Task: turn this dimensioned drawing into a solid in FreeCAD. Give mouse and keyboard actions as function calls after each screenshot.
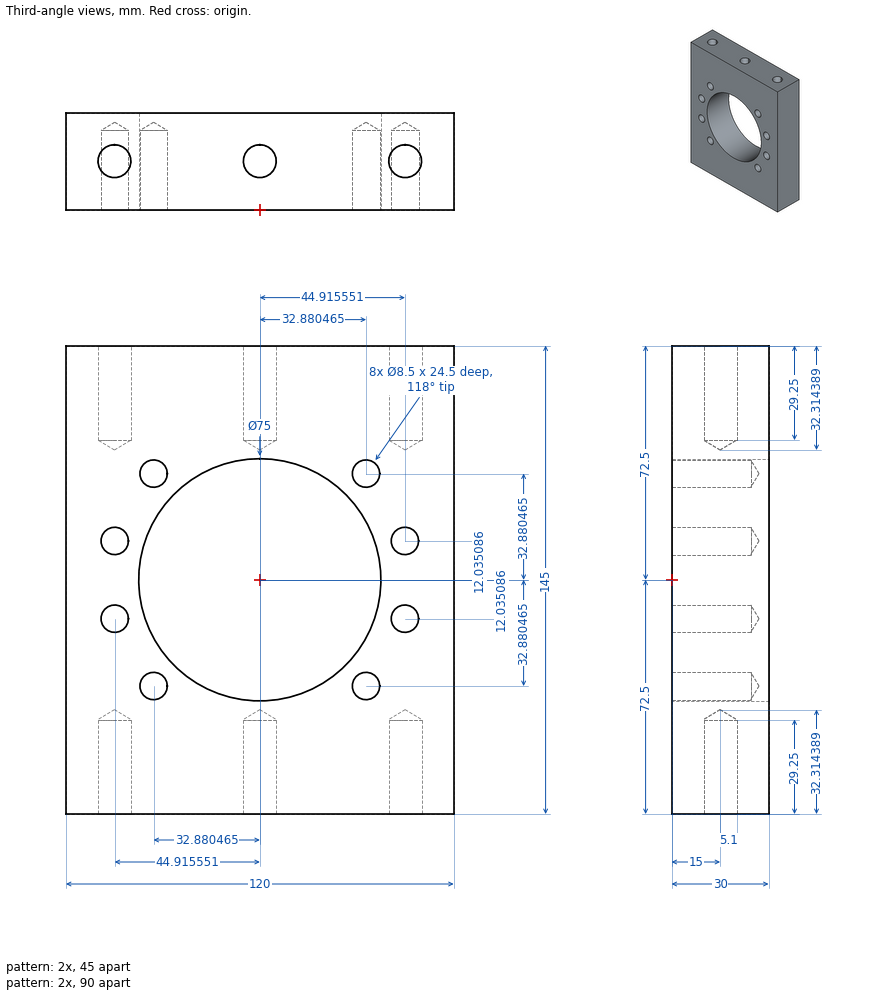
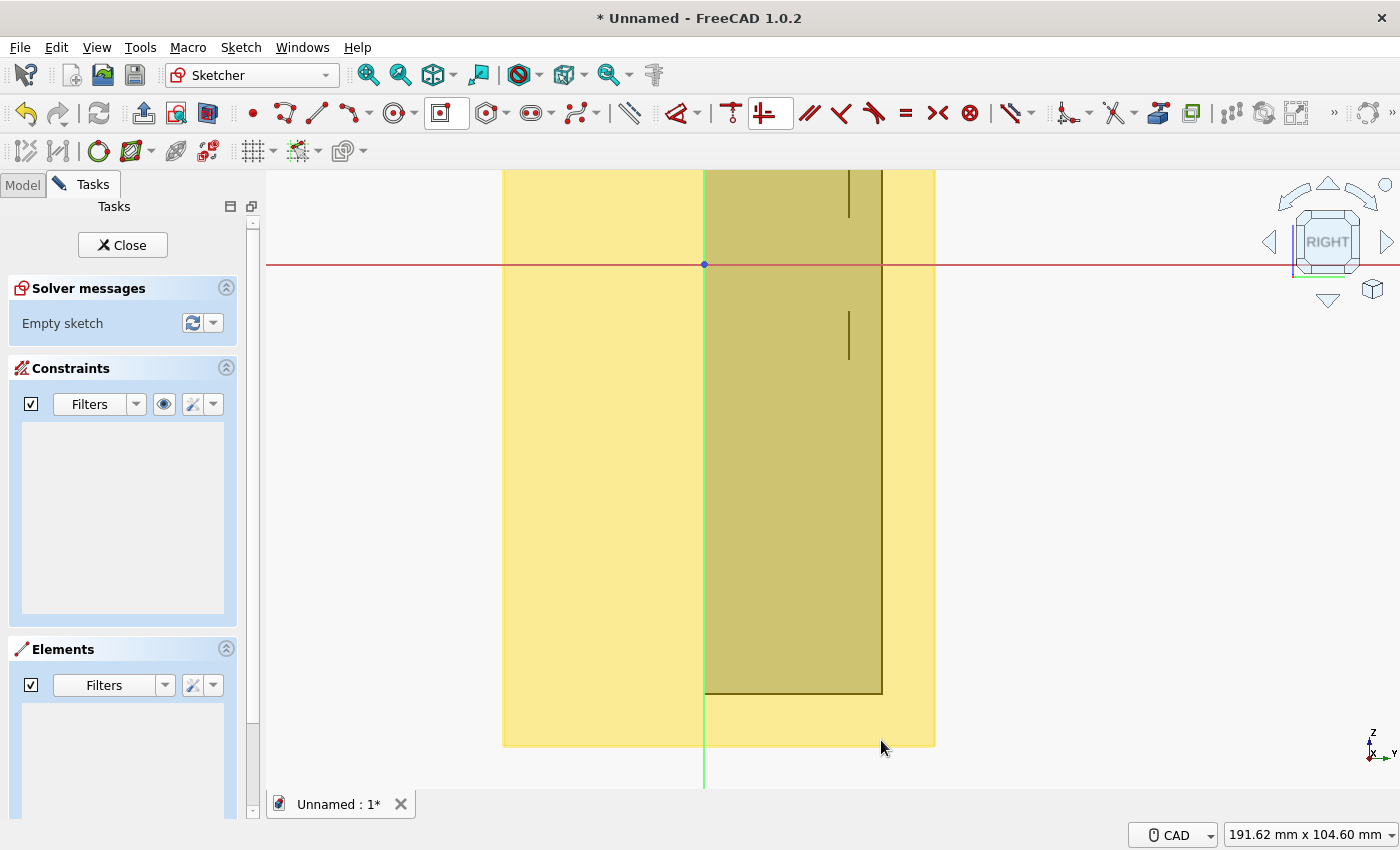
click(286, 114)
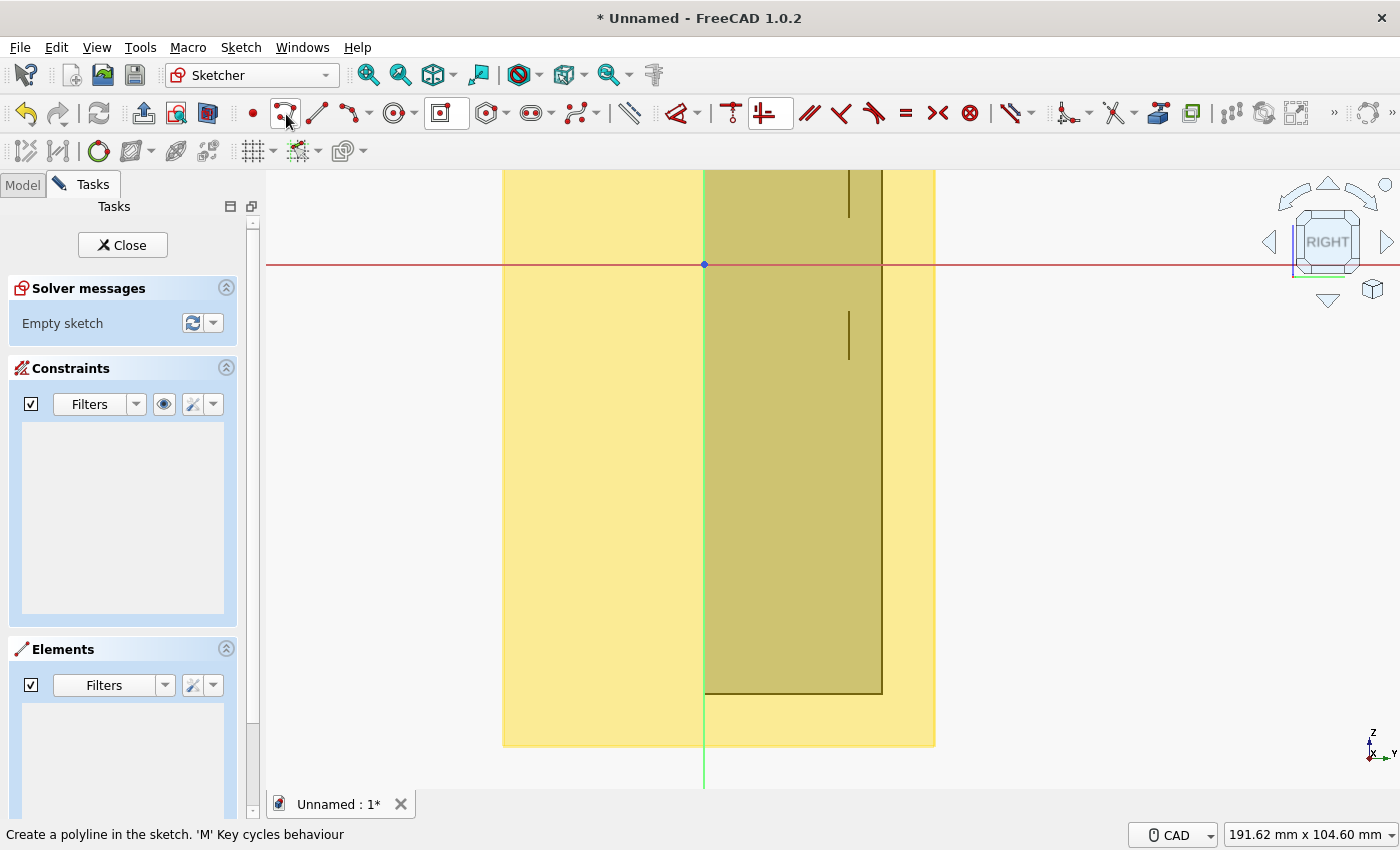
click(793, 502)
click(793, 694)
click(823, 694)
click(823, 521)
click(793, 503)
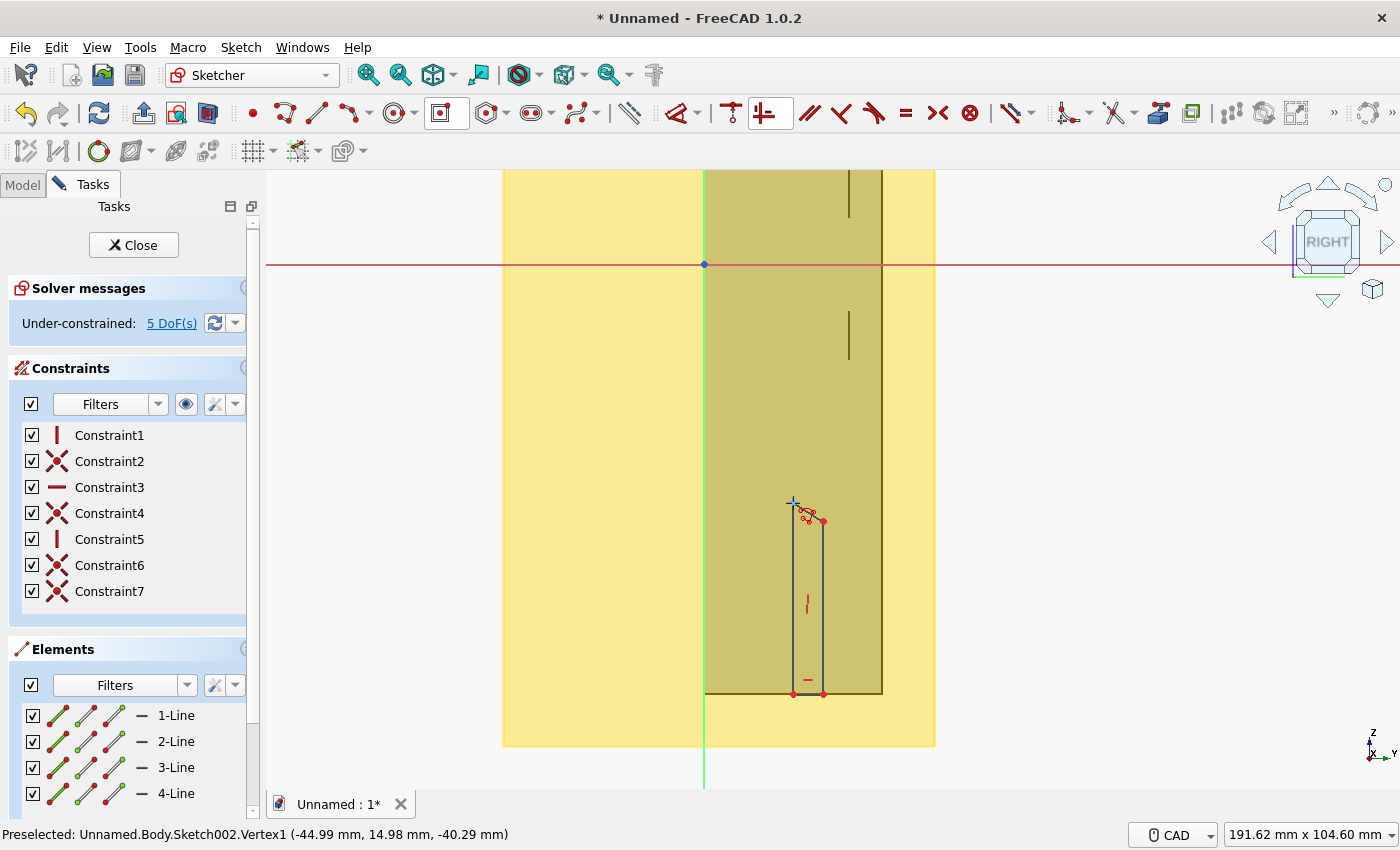
click(318, 114)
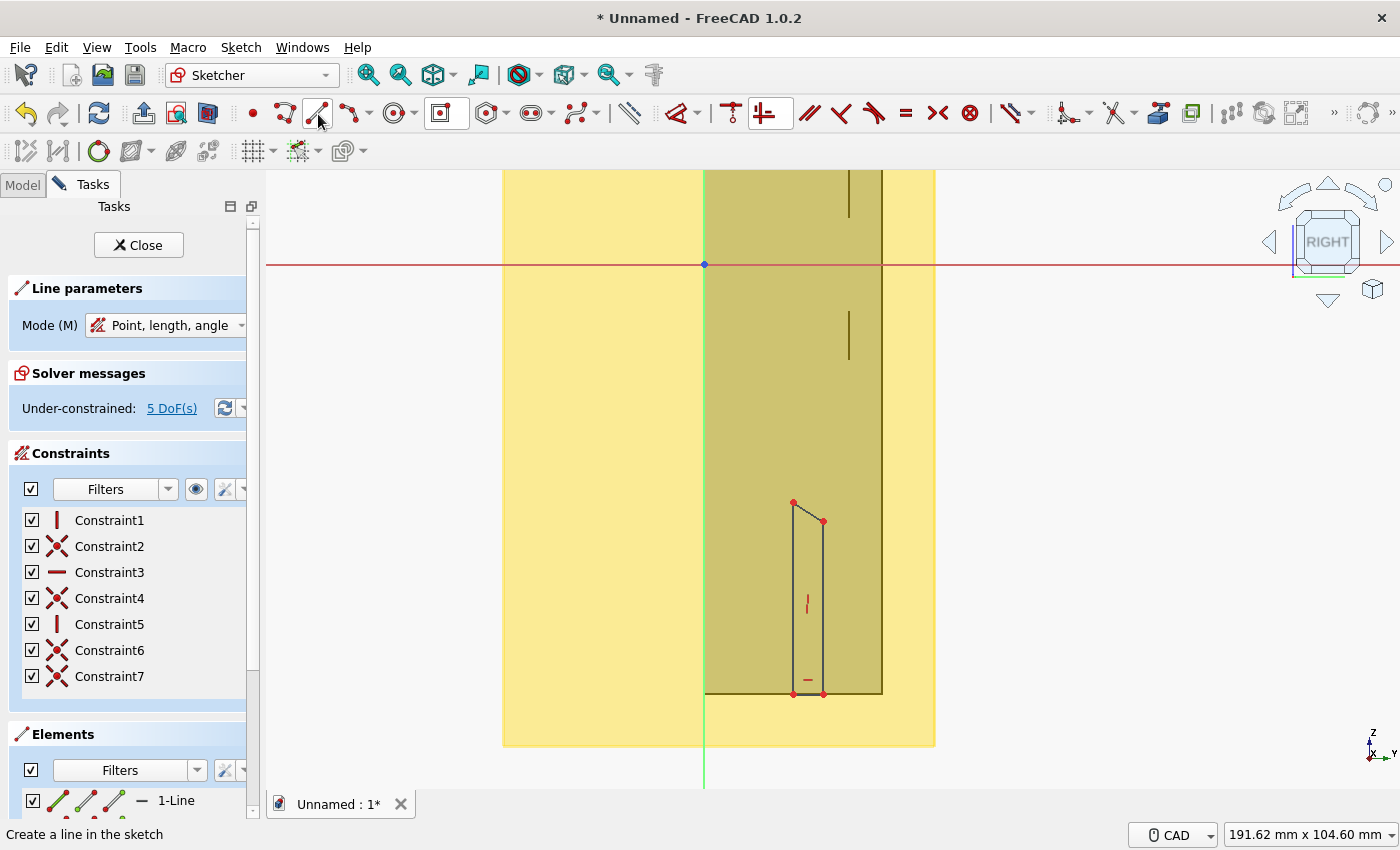
click(793, 483)
click(793, 426)
key(Escape)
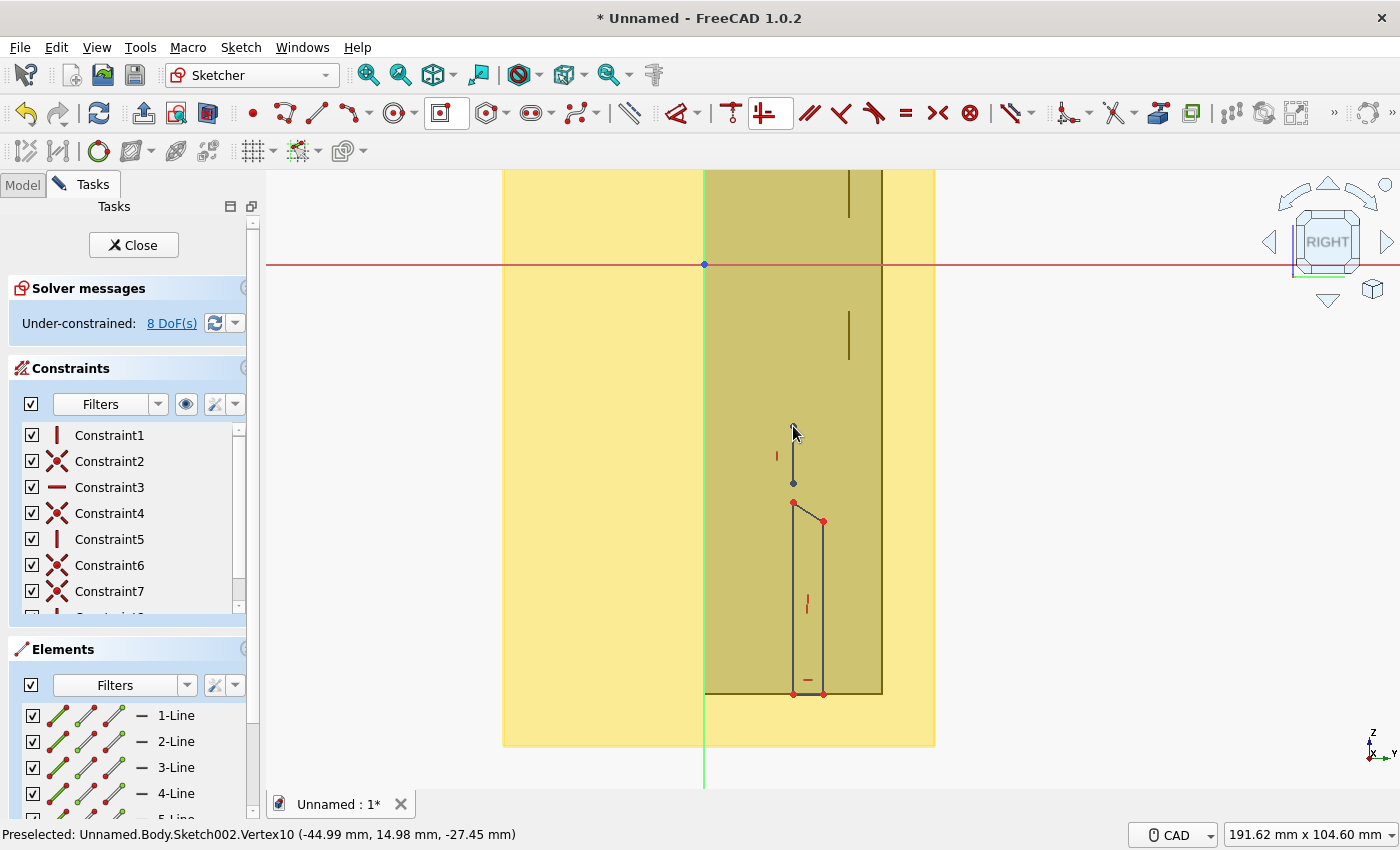
click(793, 467)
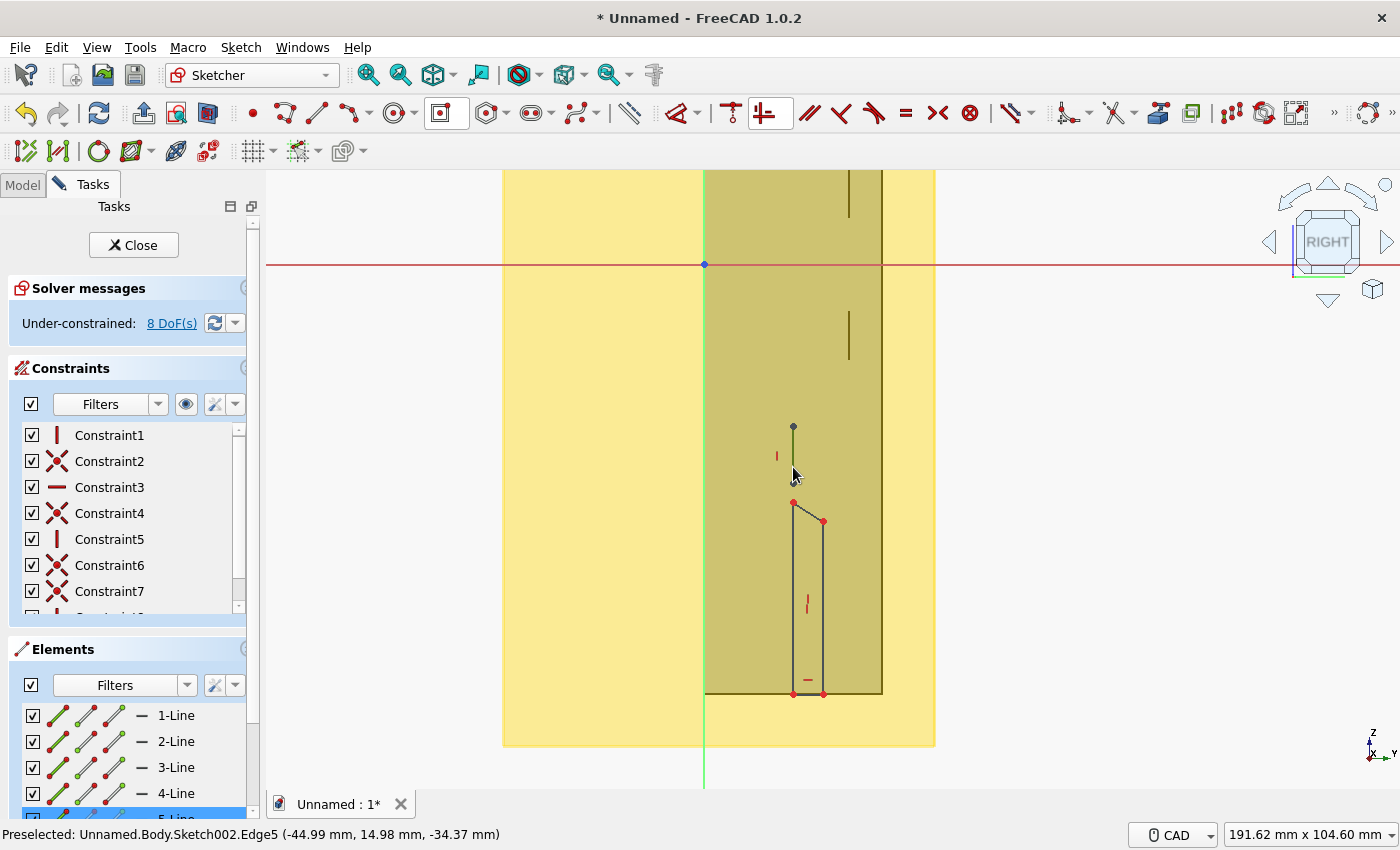
click(630, 114)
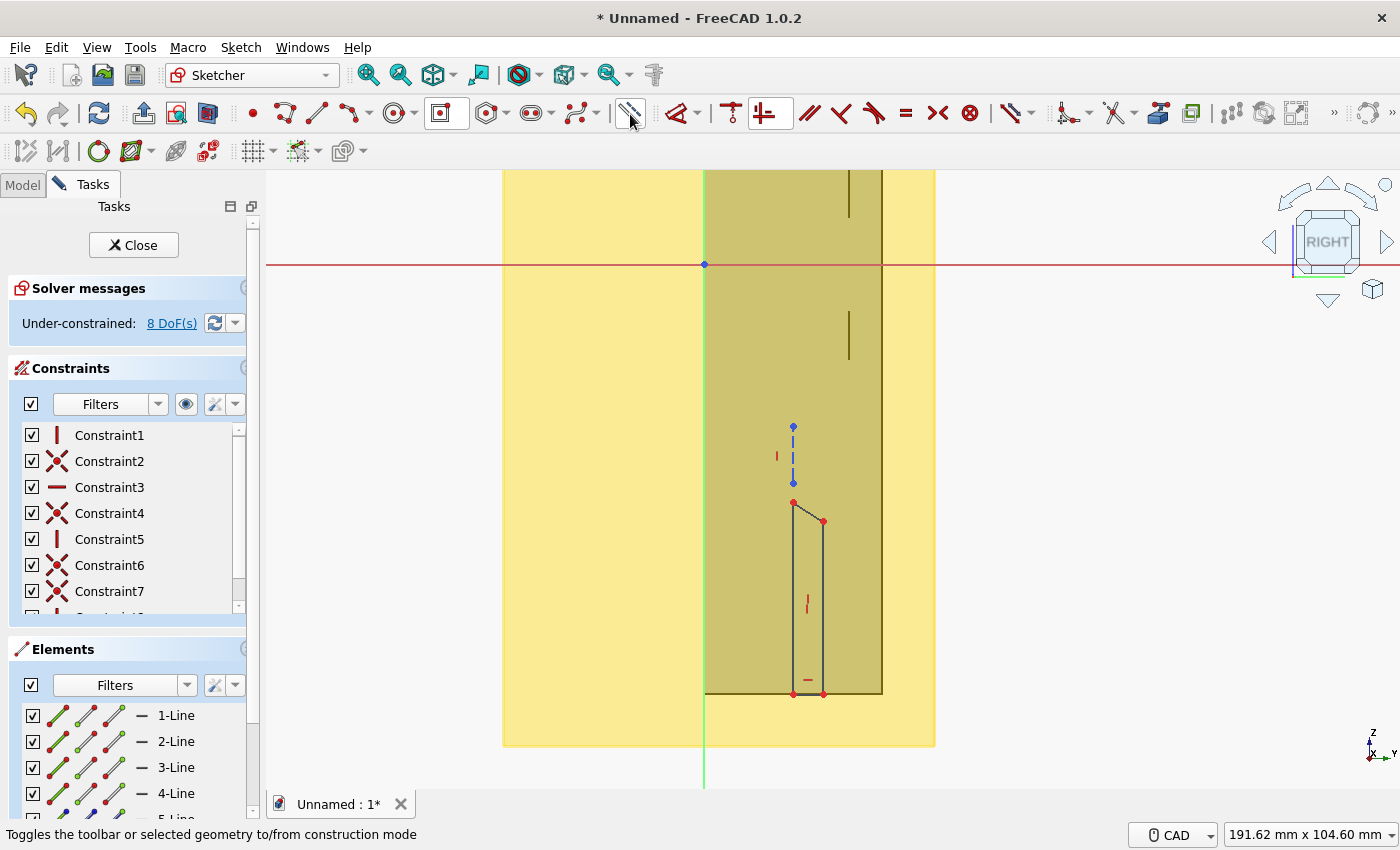
click(676, 114)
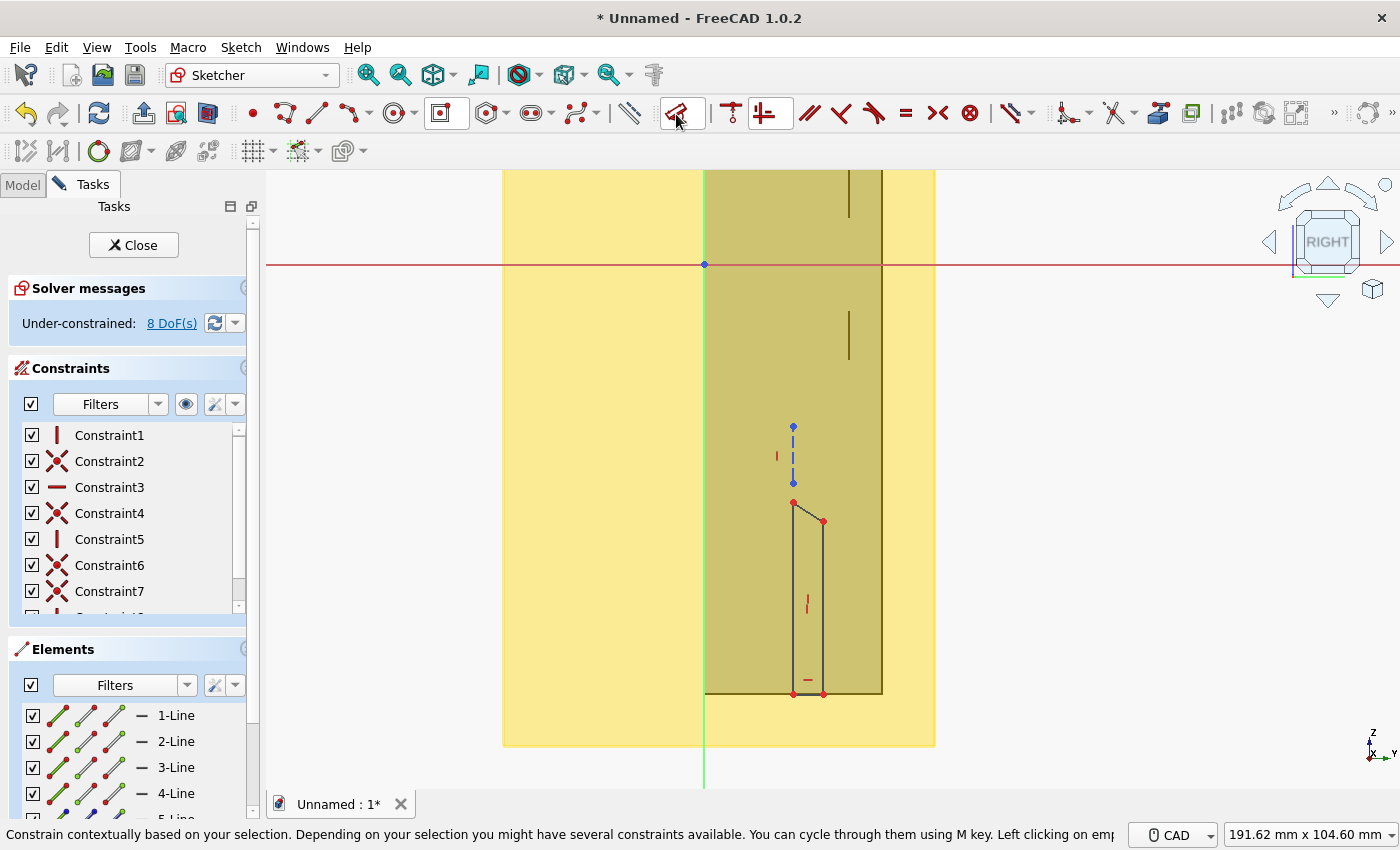
scroll(802, 695, up, 3)